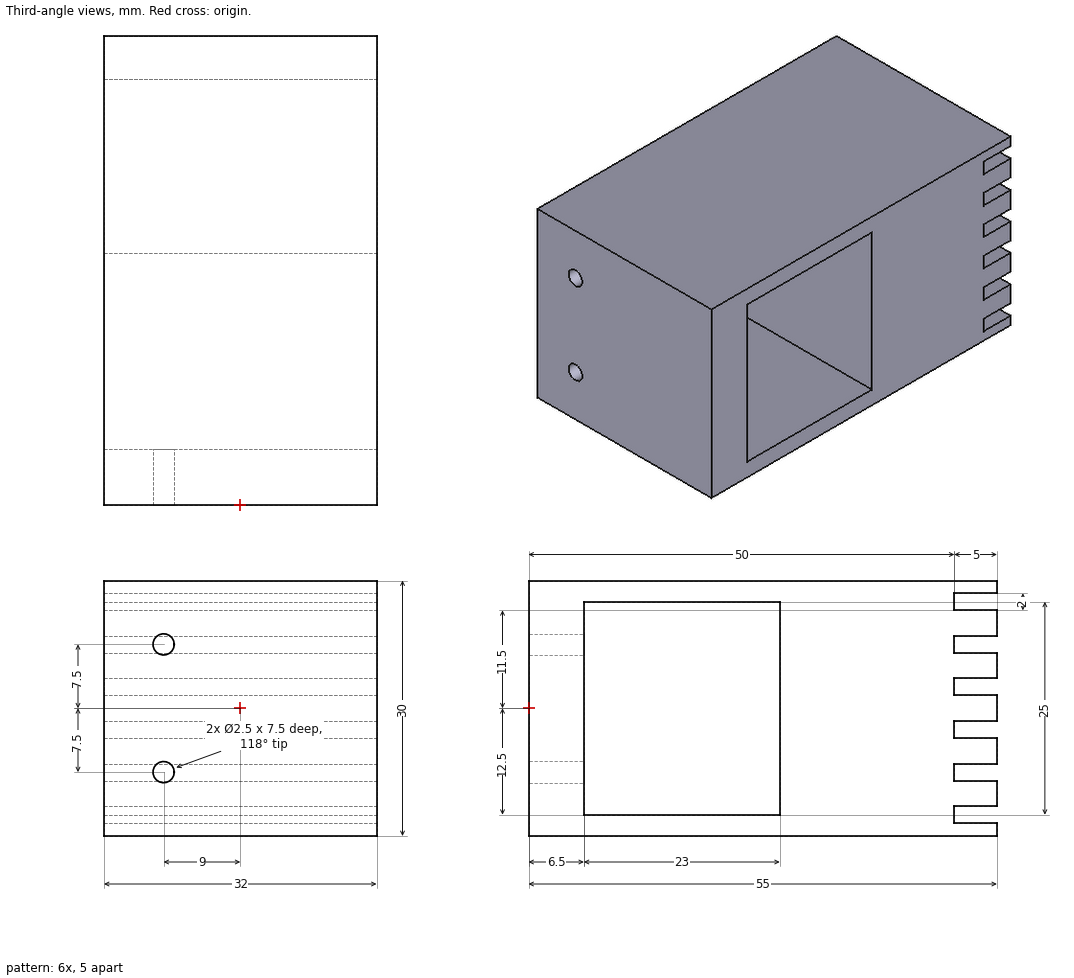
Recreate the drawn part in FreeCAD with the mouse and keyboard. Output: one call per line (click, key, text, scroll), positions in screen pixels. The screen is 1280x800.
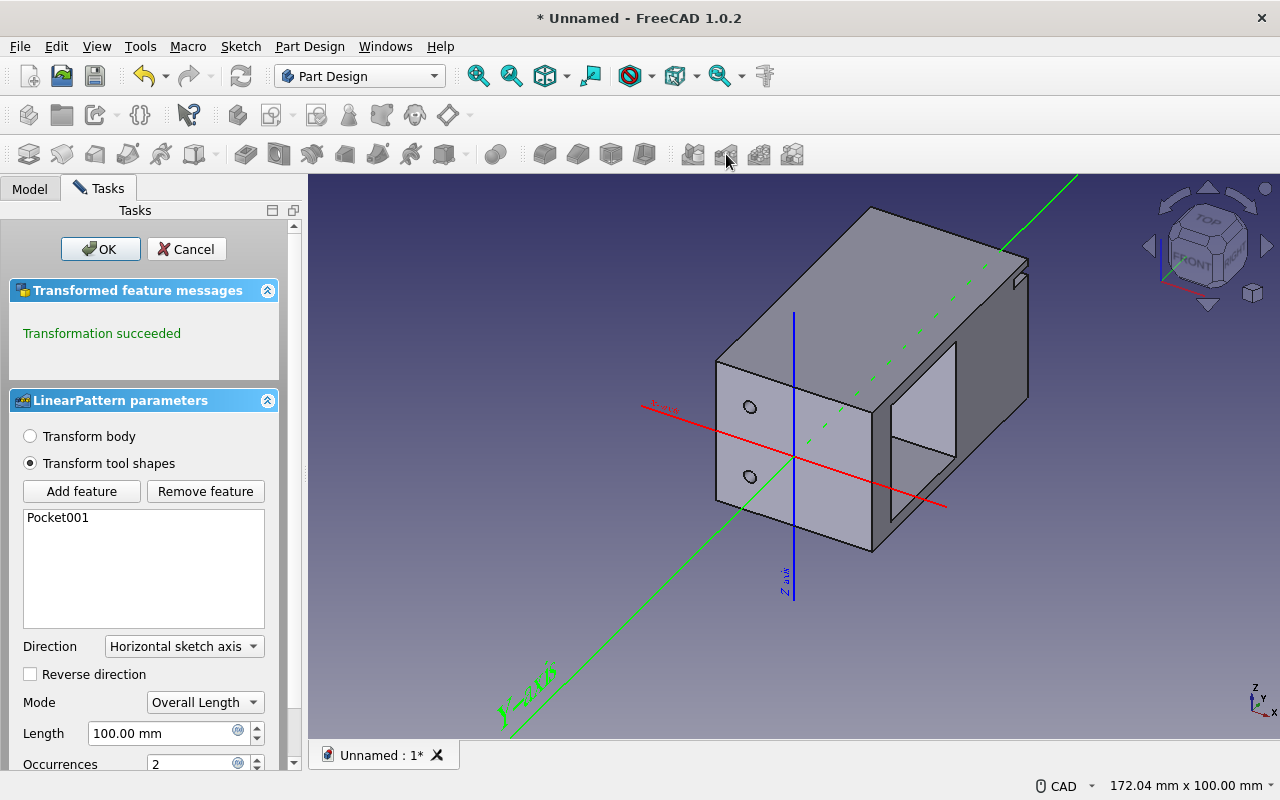
click(185, 646)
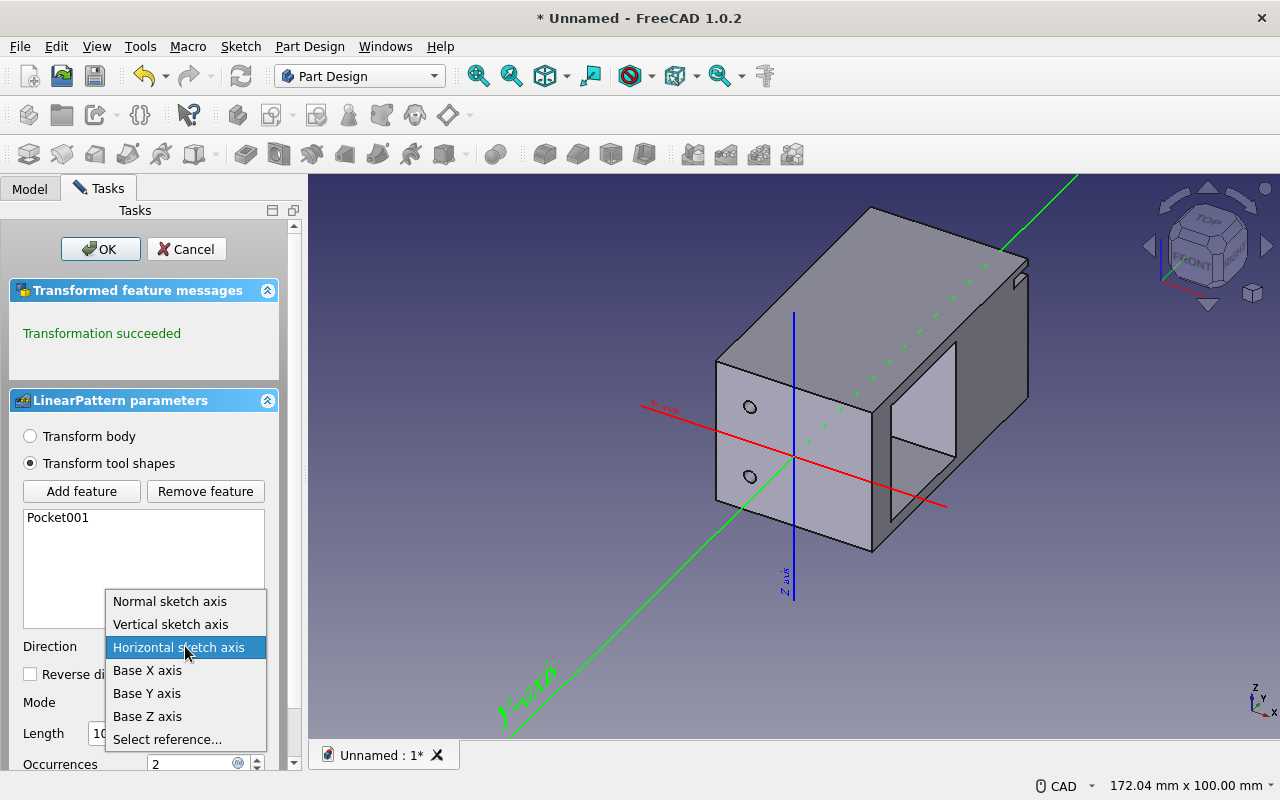
click(184, 716)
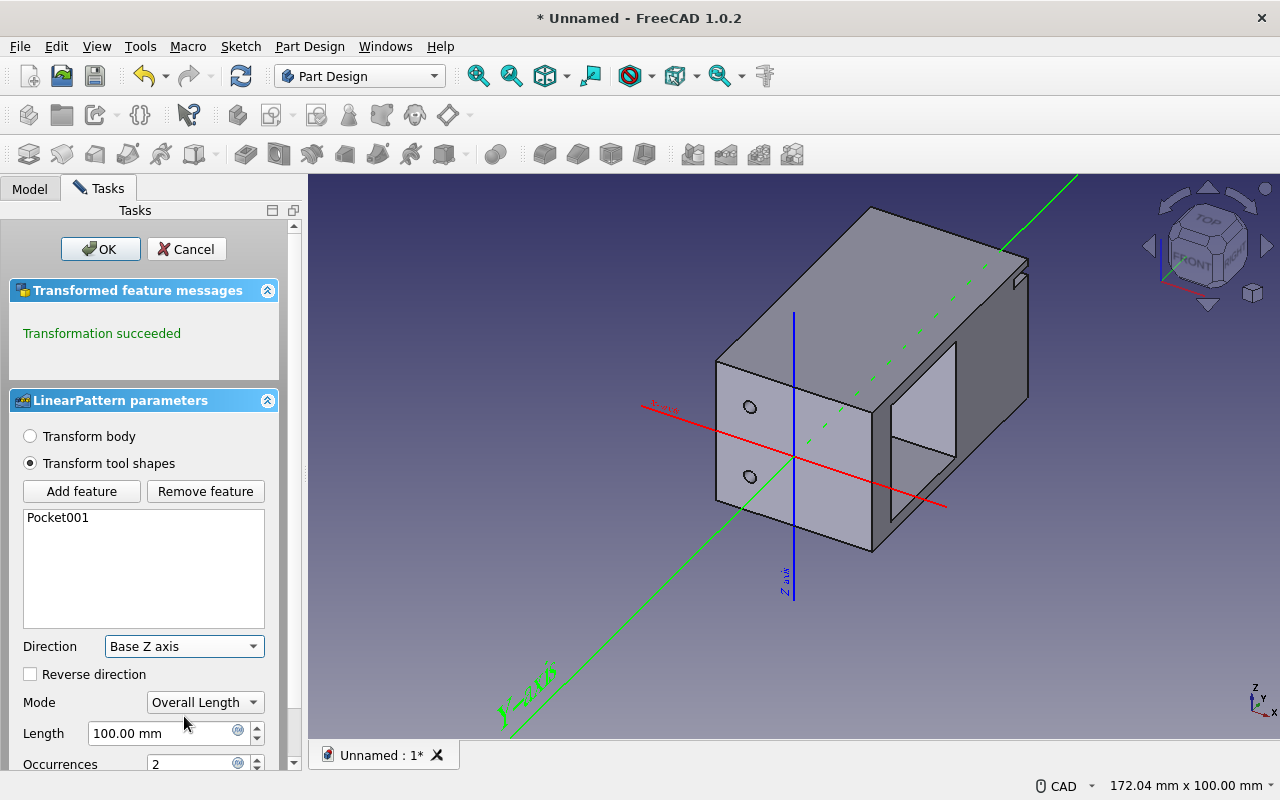
click(206, 702)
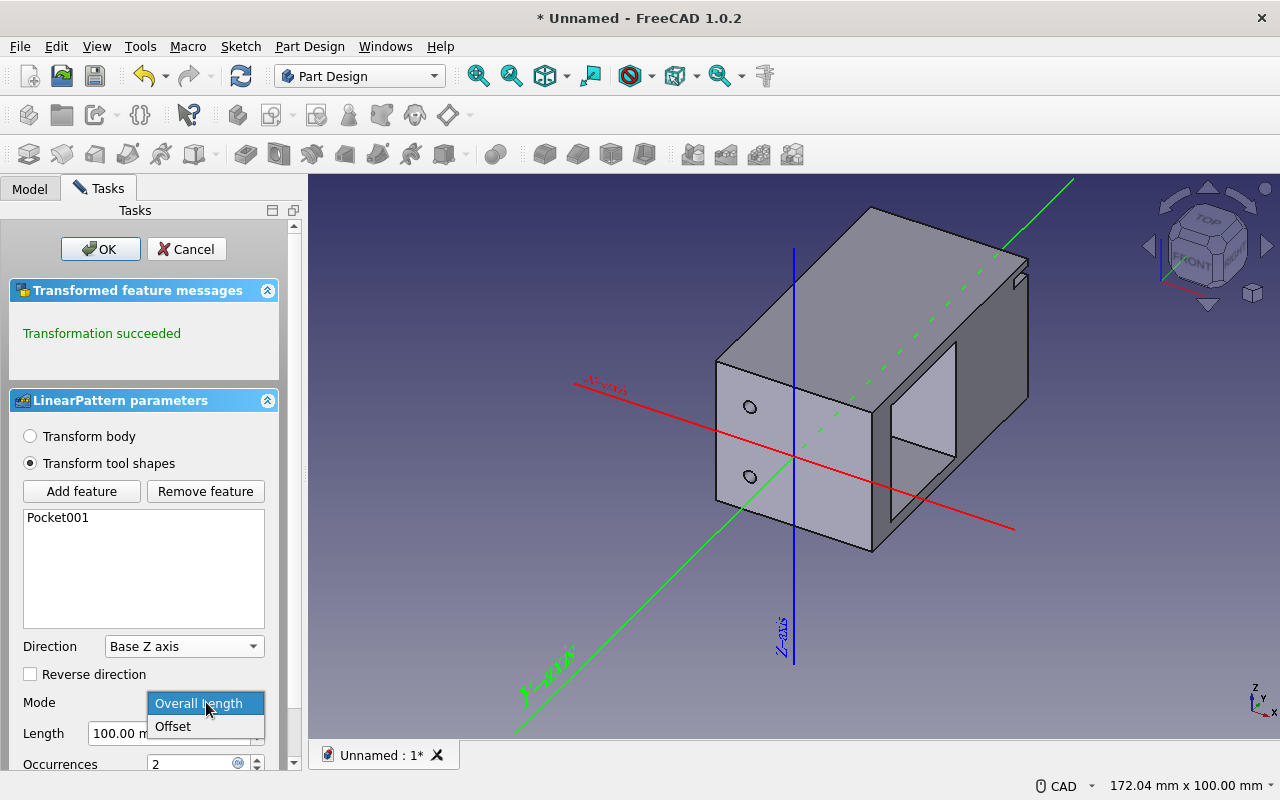
click(204, 726)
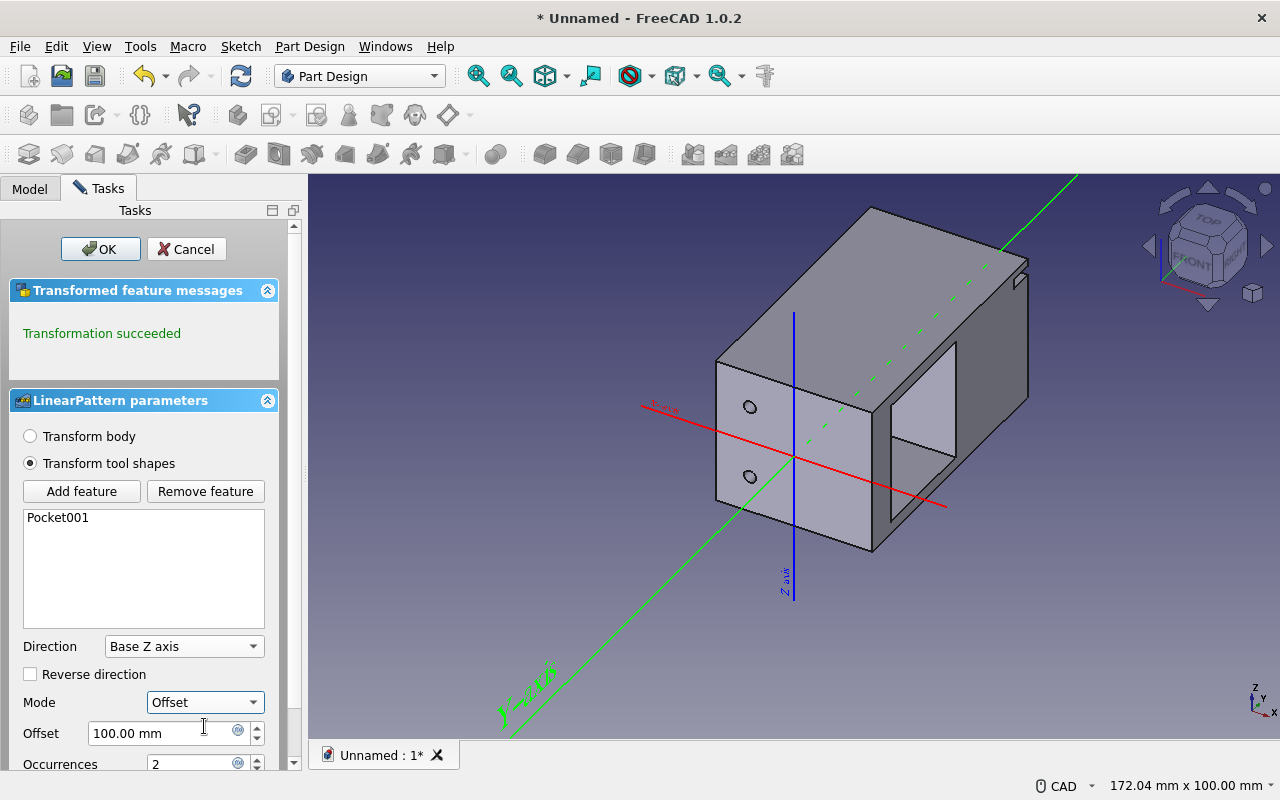
triple_click(170, 734)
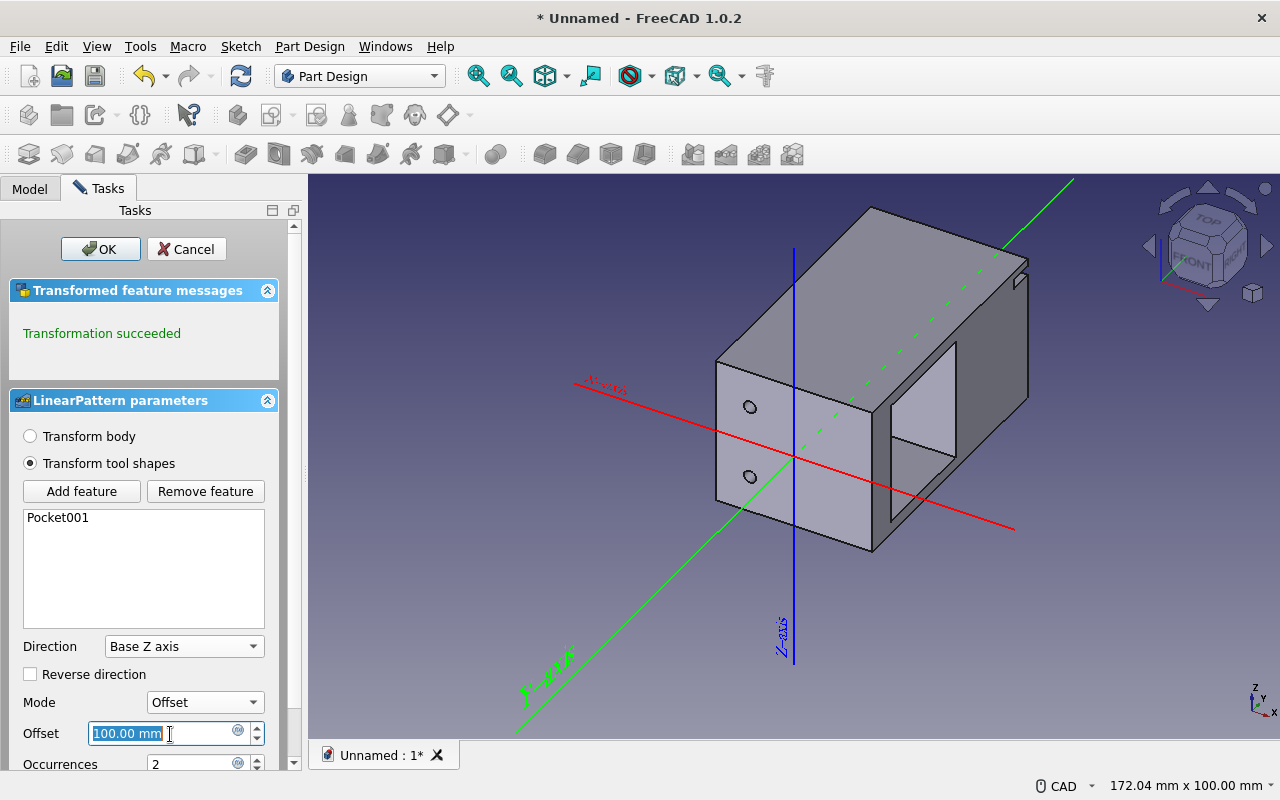
text(5)
key(Tab)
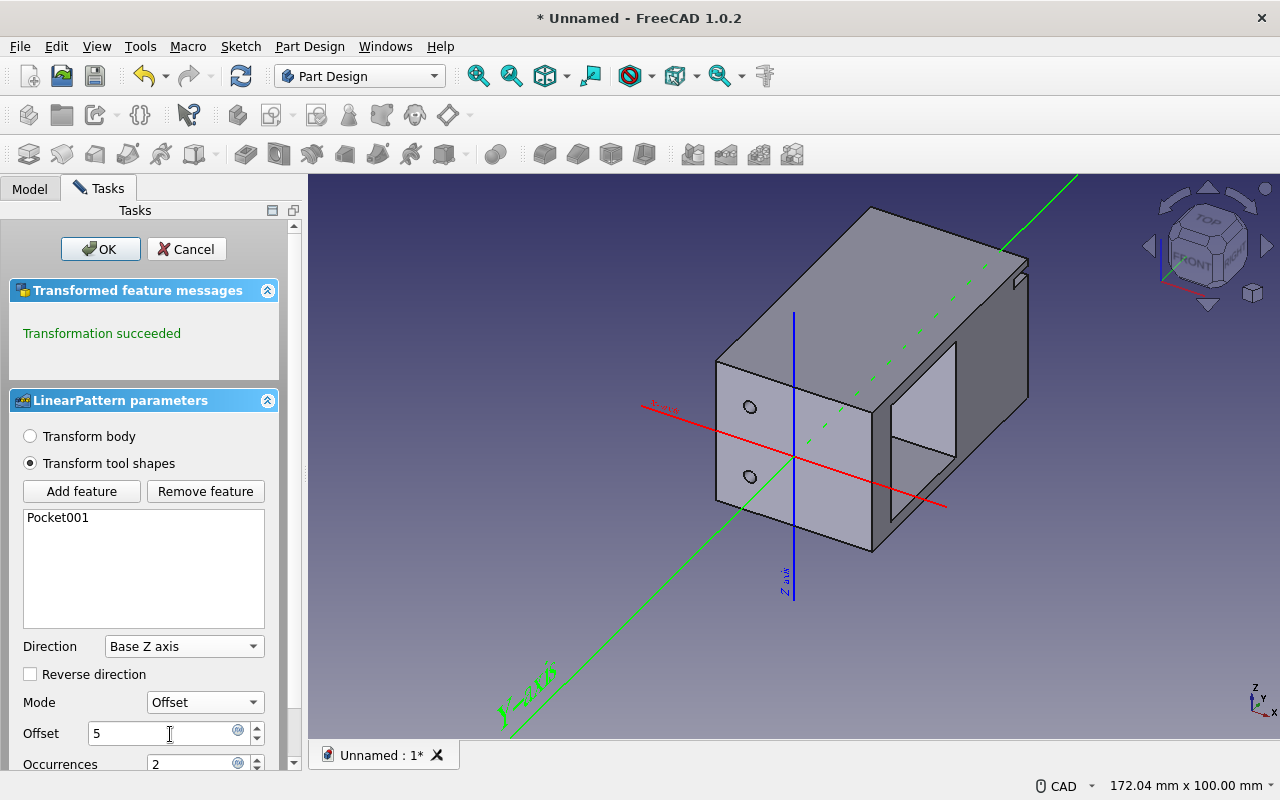
scroll(294, 495, down, 2)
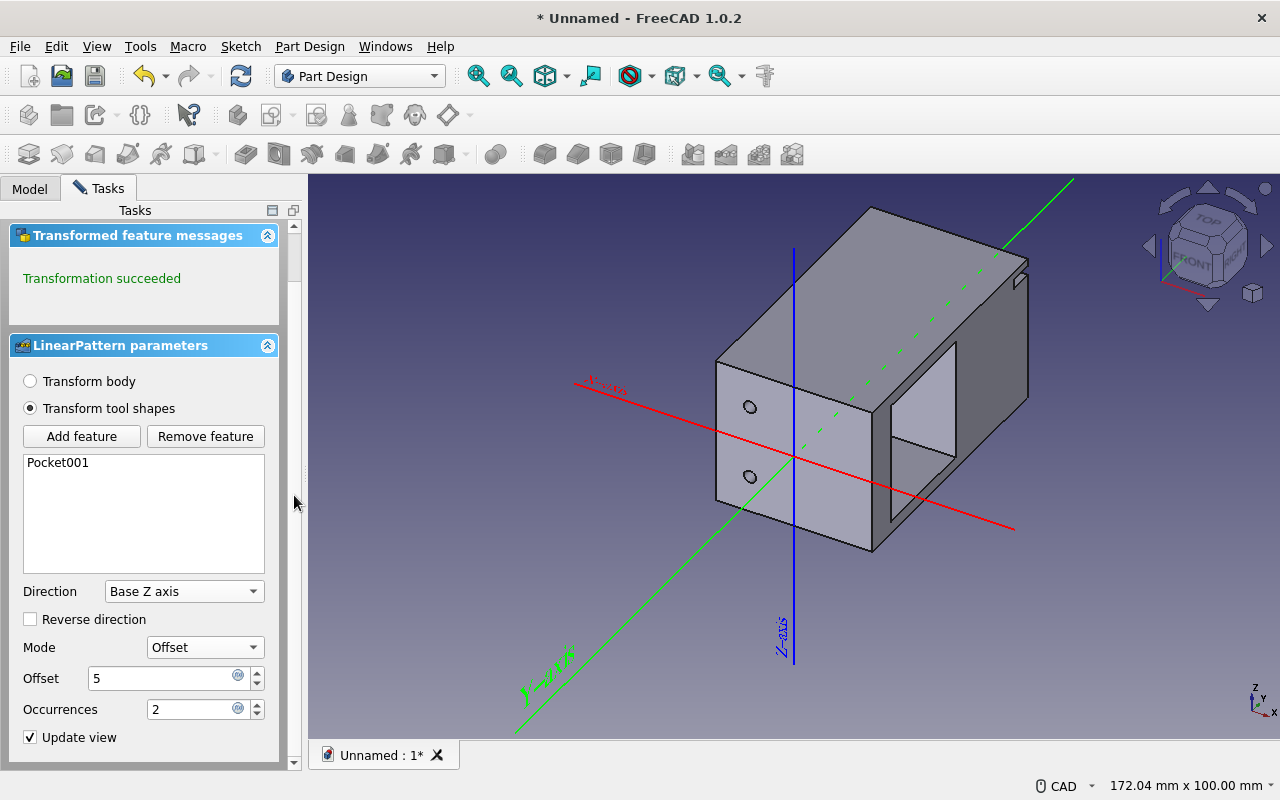
triple_click(199, 710)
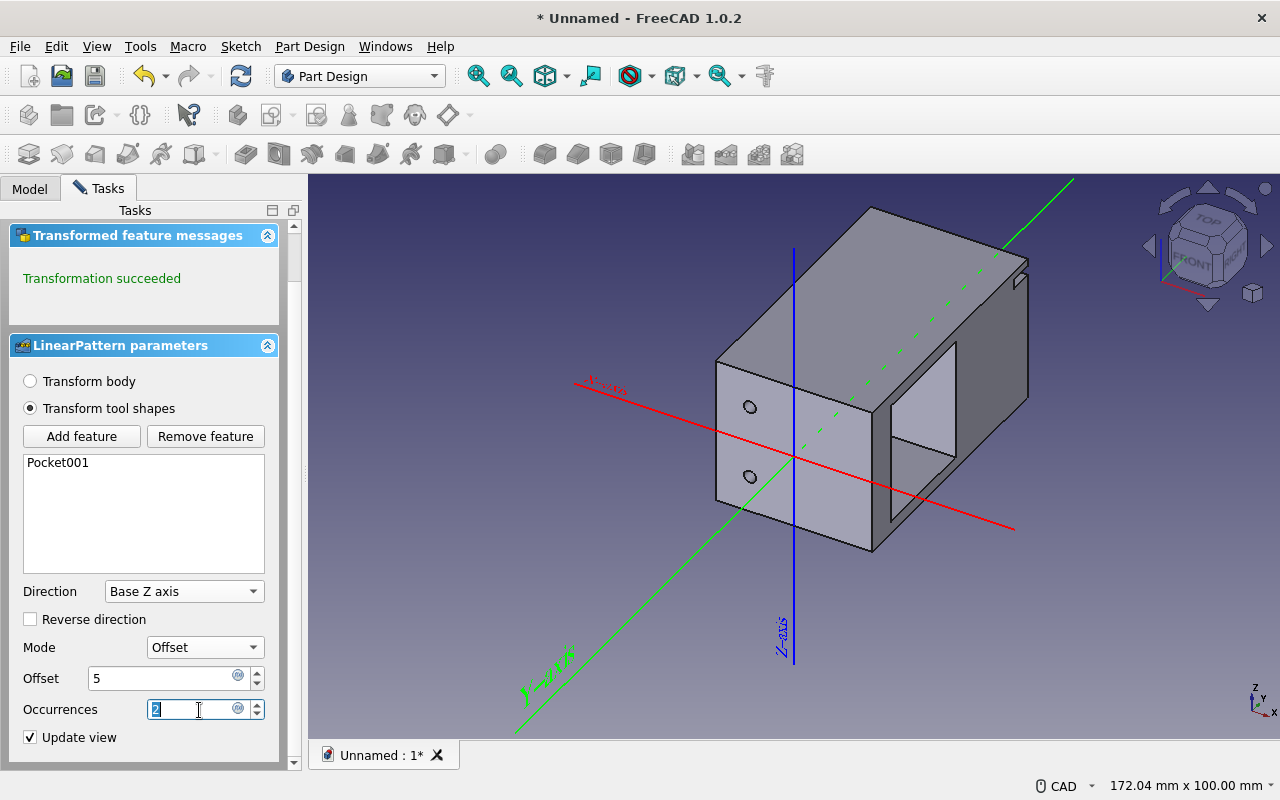
text(6)
key(Tab)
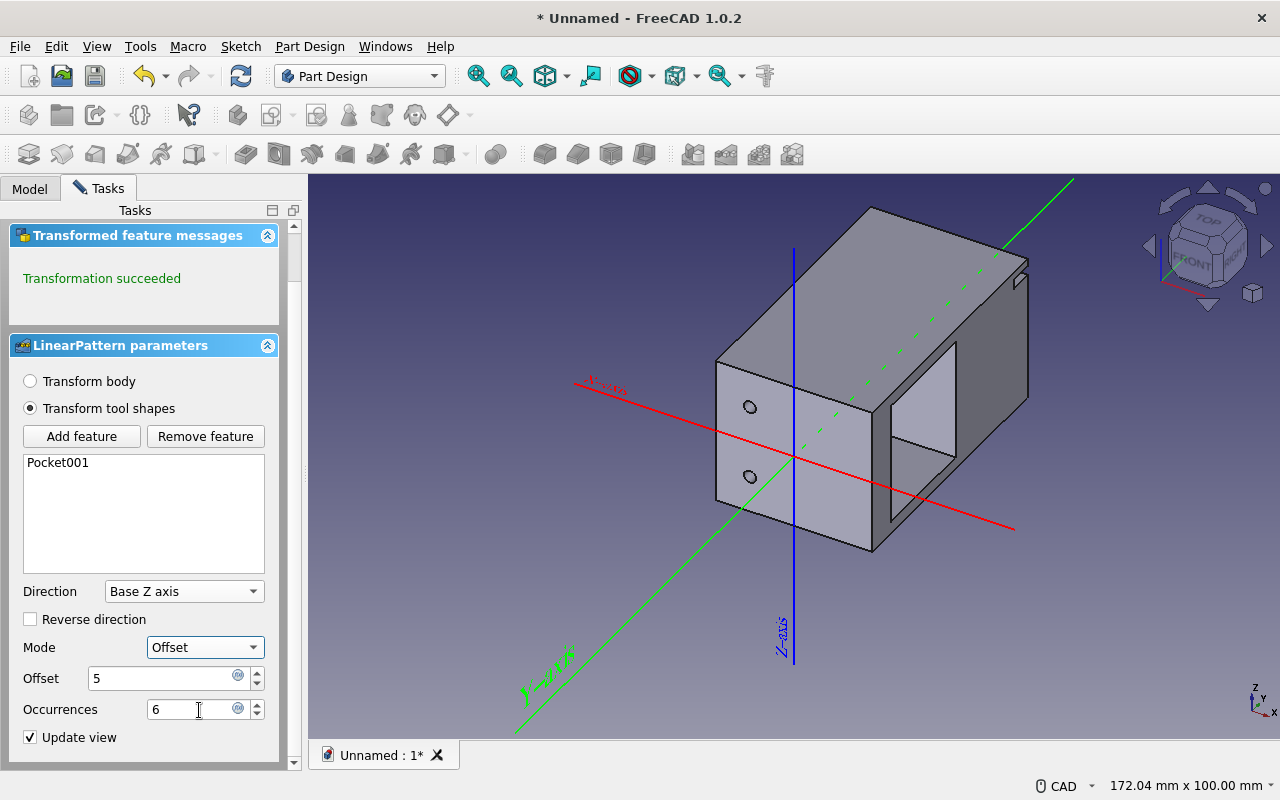
click(31, 619)